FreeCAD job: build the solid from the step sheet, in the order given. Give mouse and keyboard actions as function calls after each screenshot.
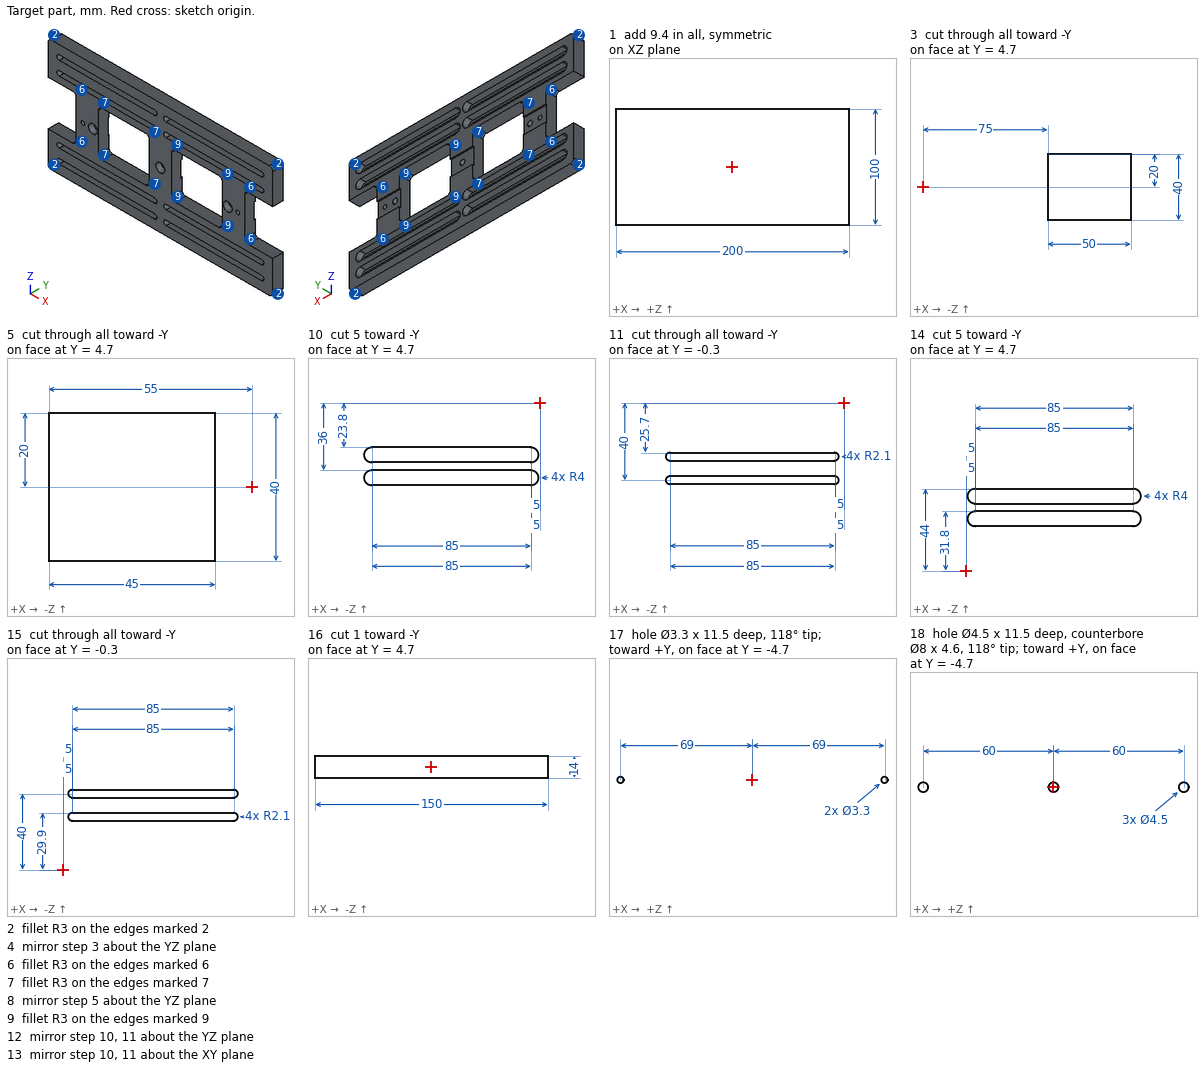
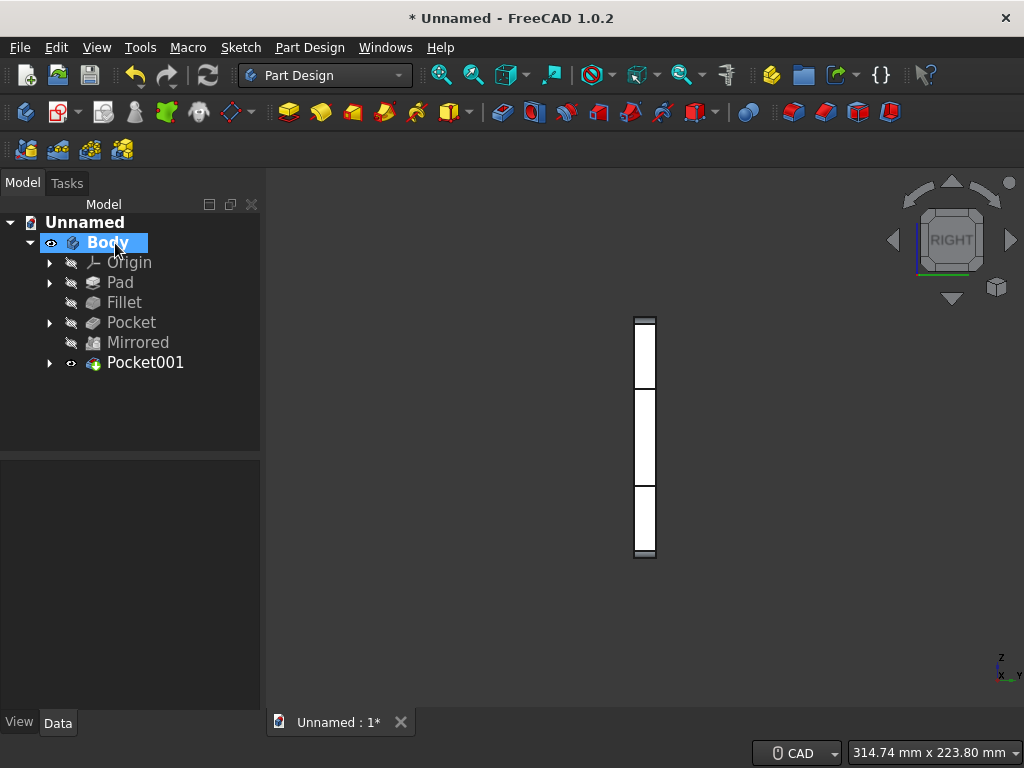
key(5)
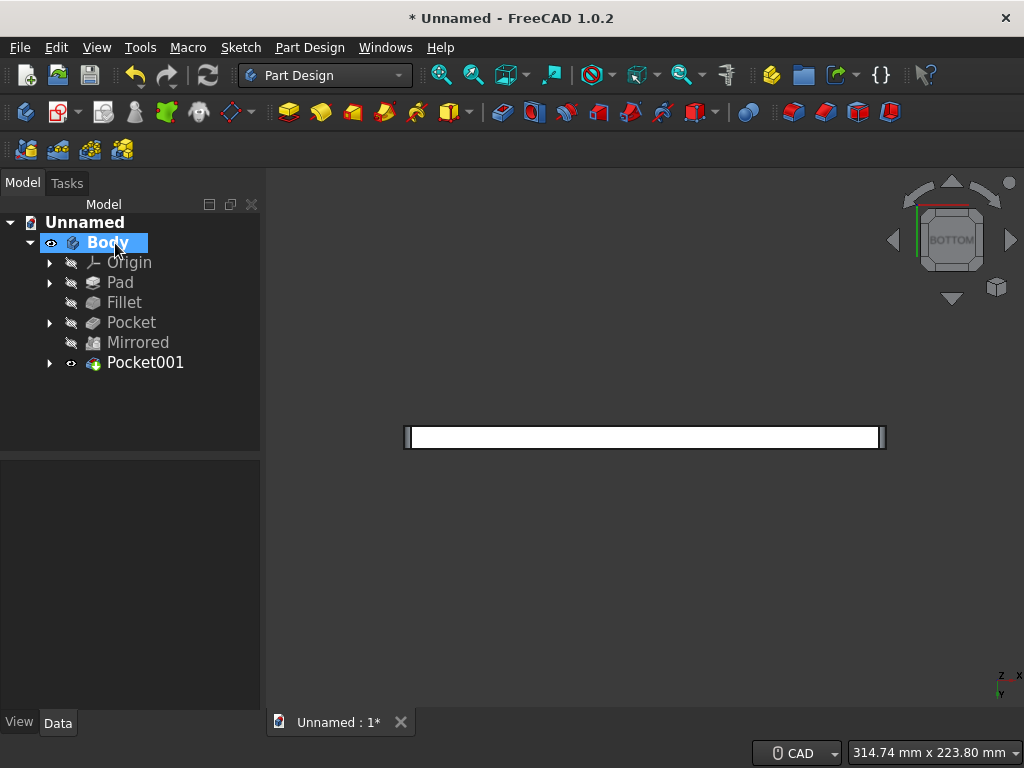
key(4)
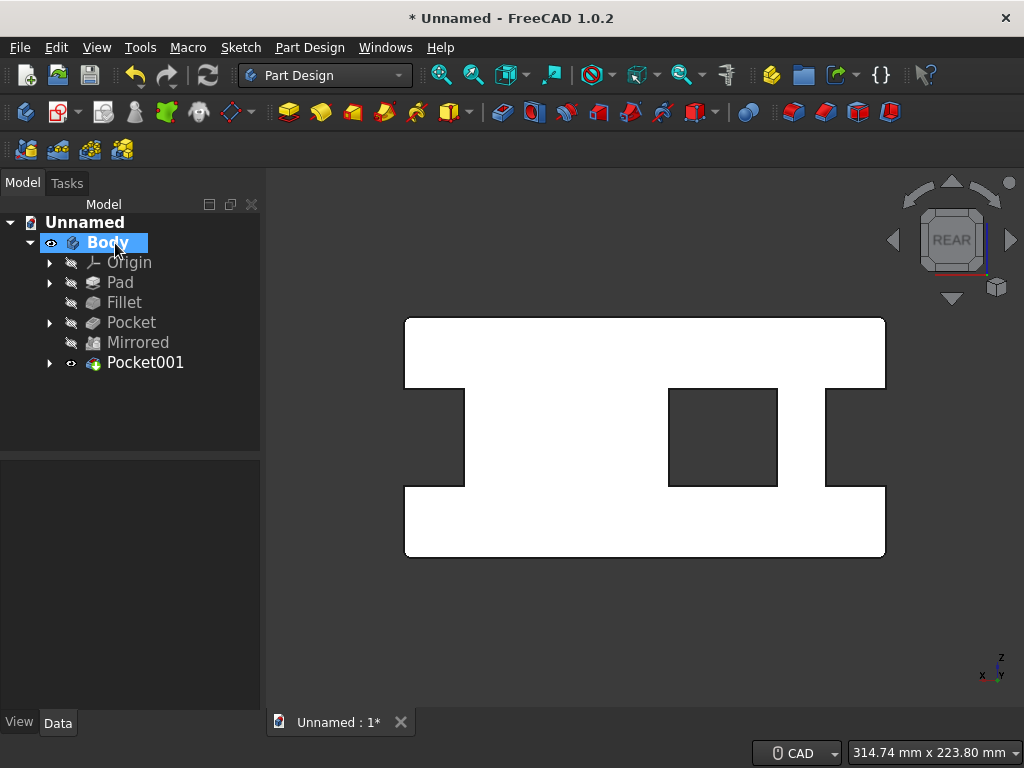
key(6)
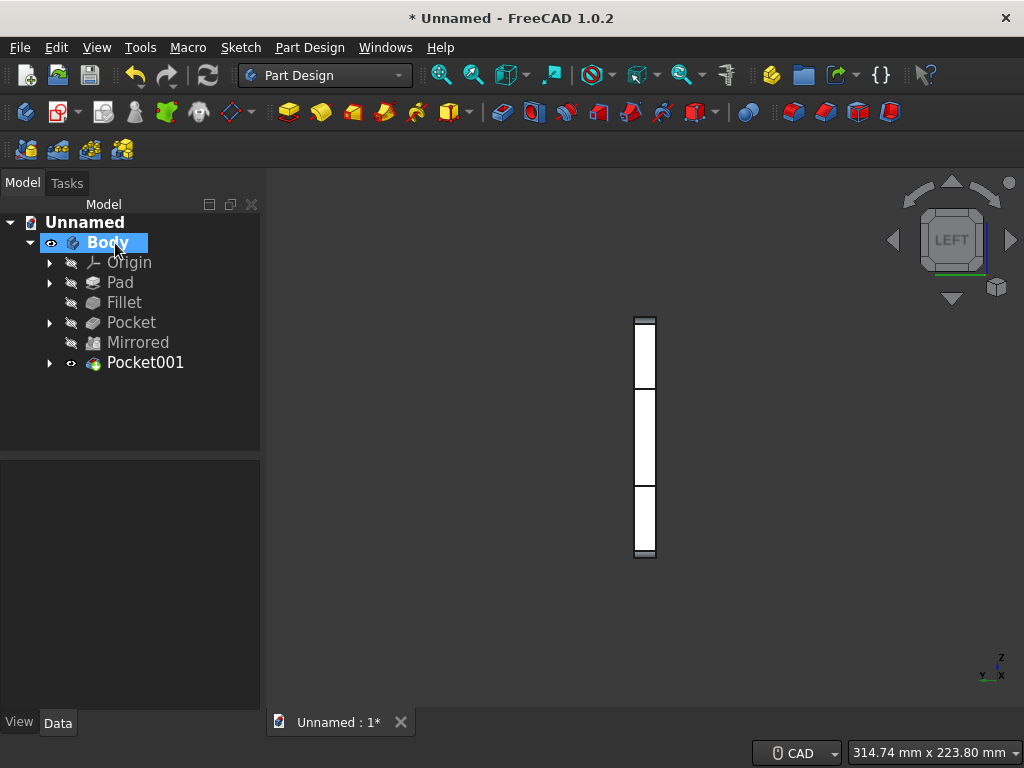
click(442, 76)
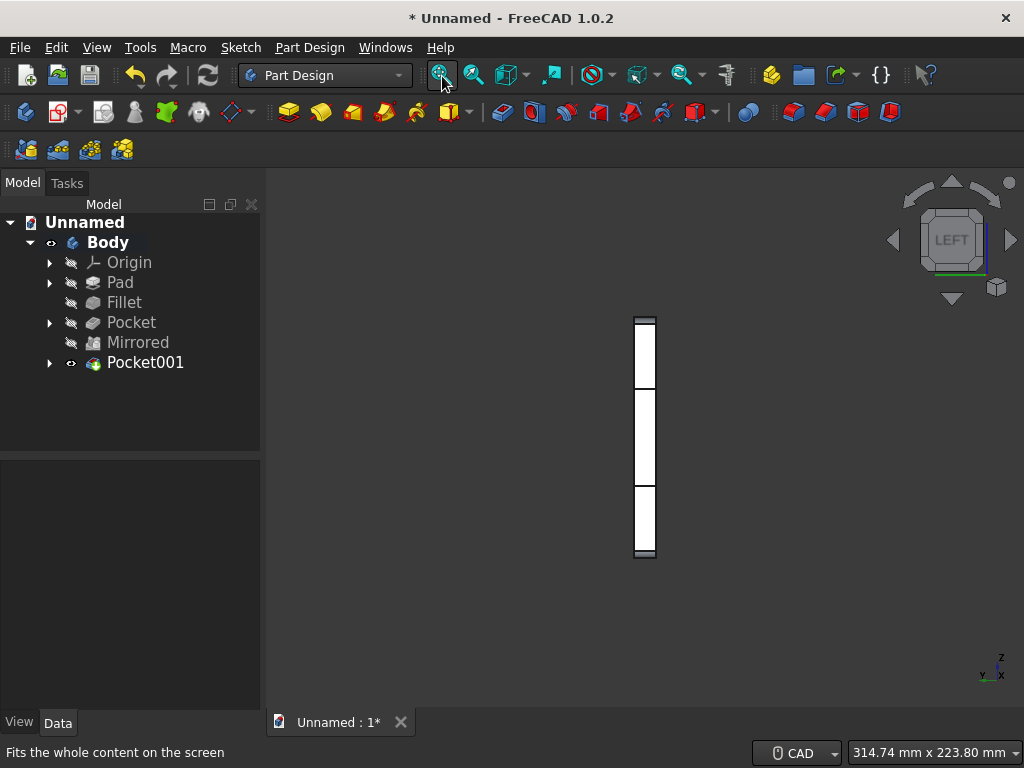
key(v)
key(3)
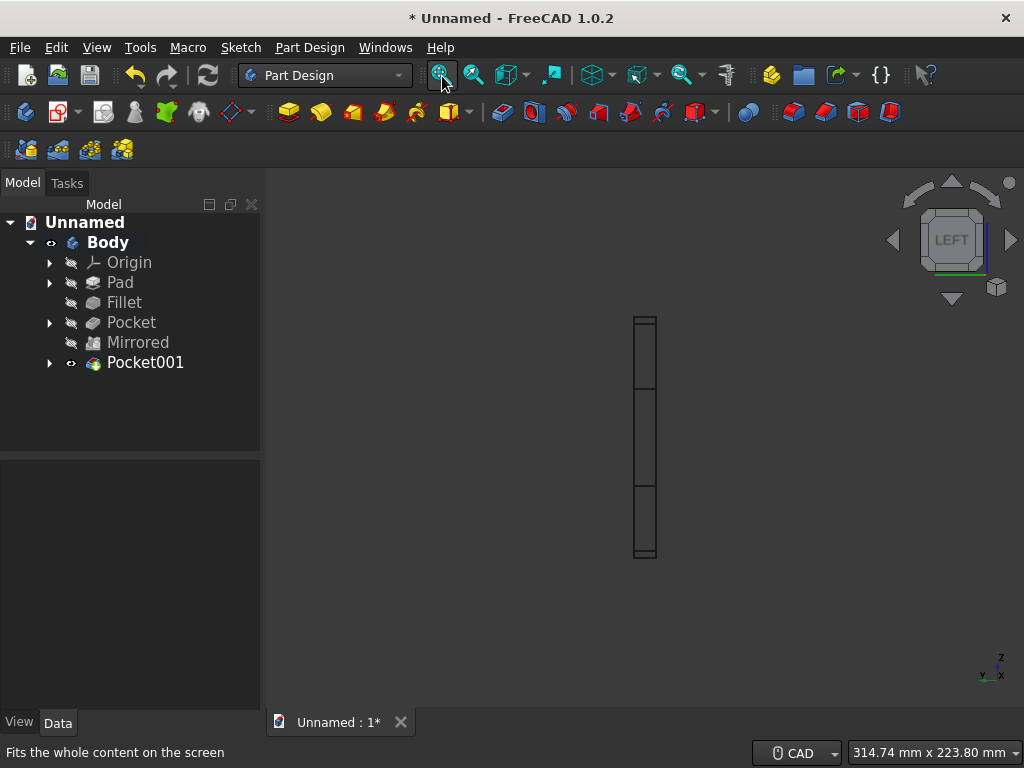
key(0)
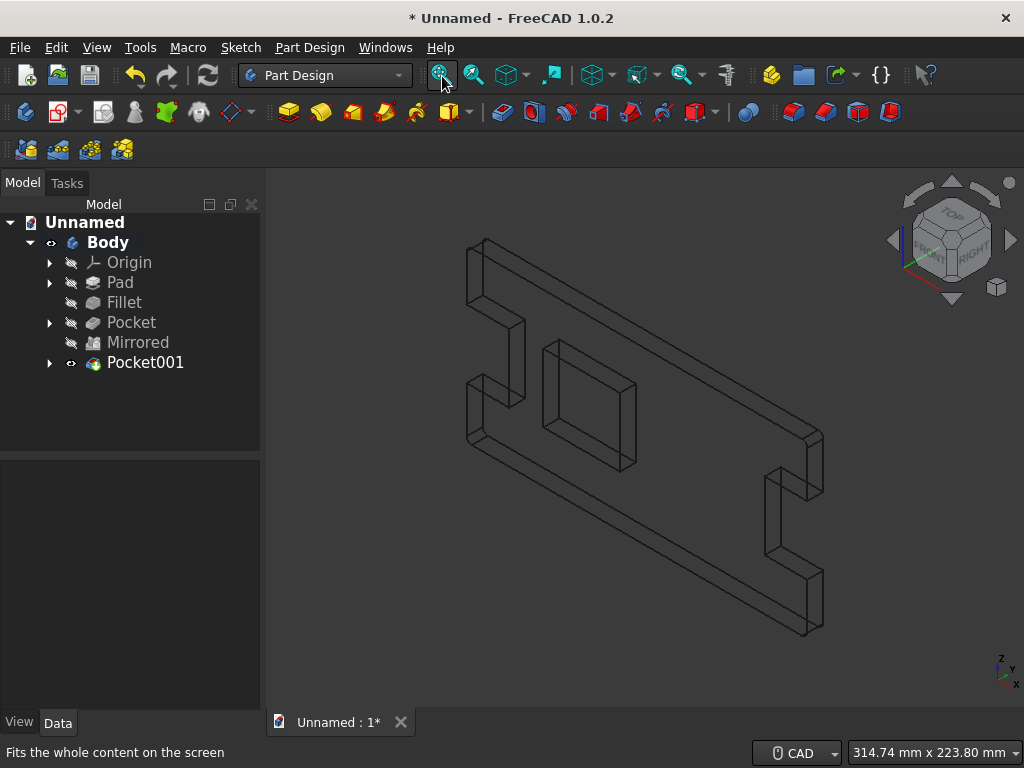
click(773, 550)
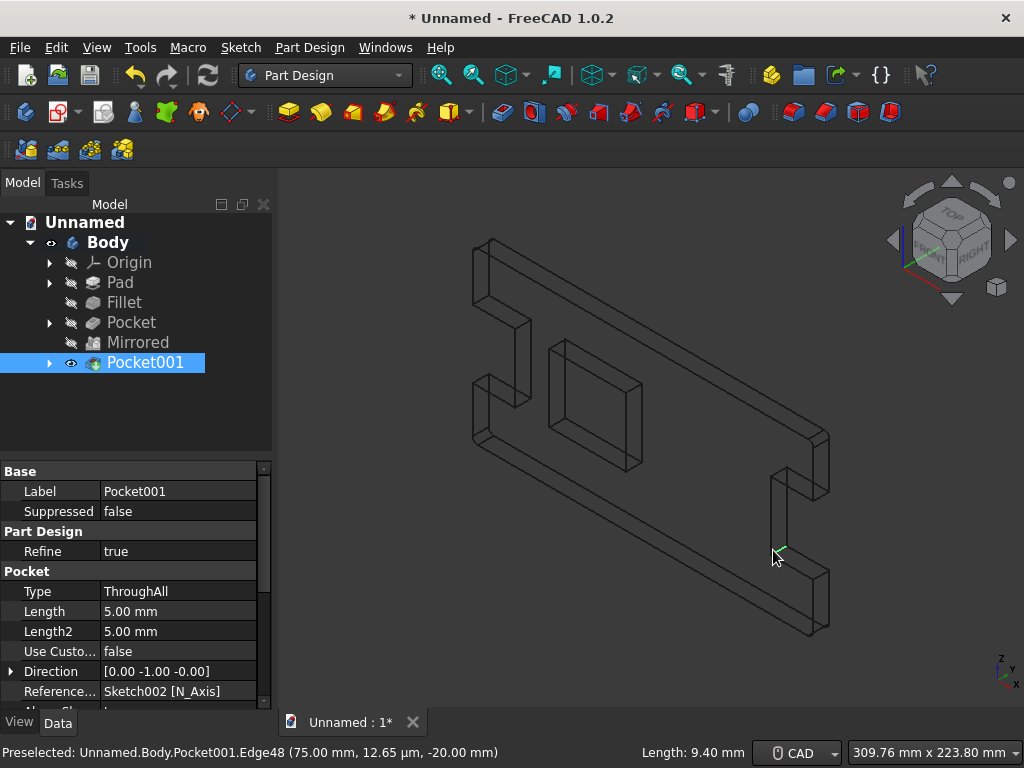
click(779, 471, ctrl)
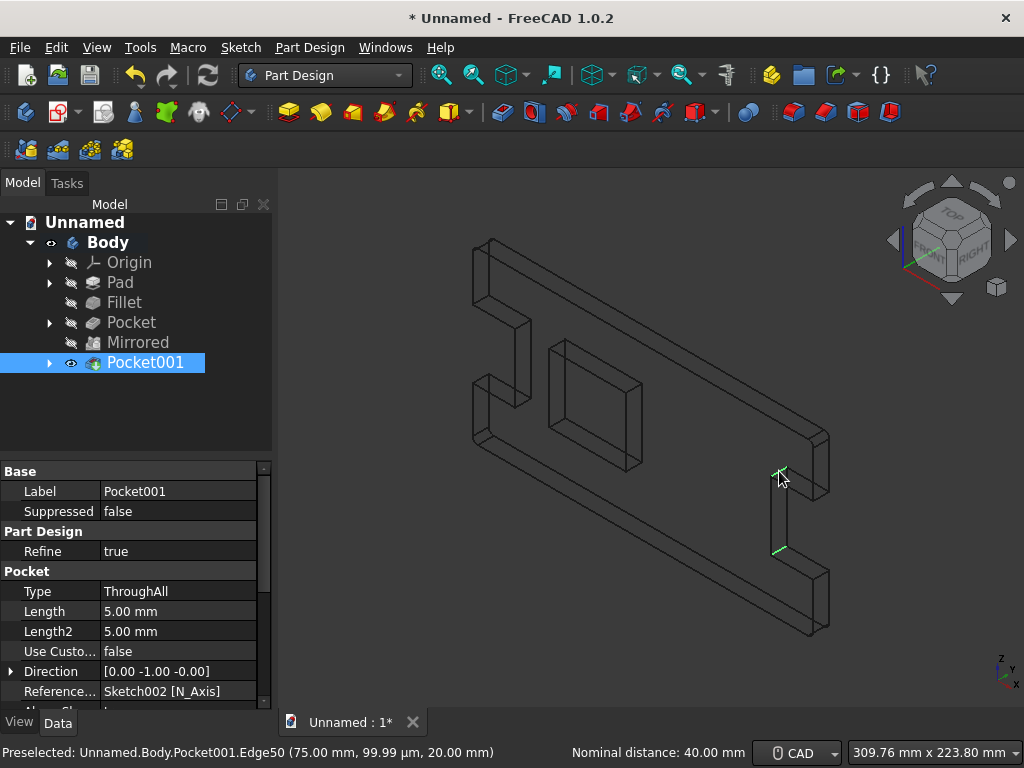
click(523, 323, ctrl)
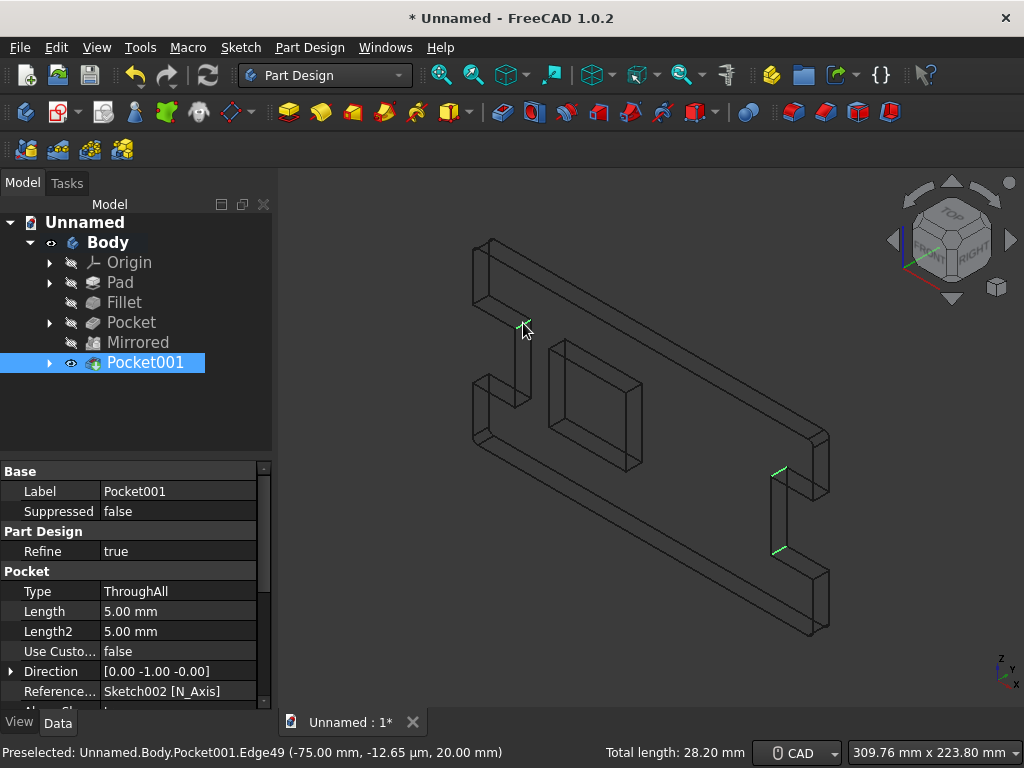
click(523, 402, ctrl)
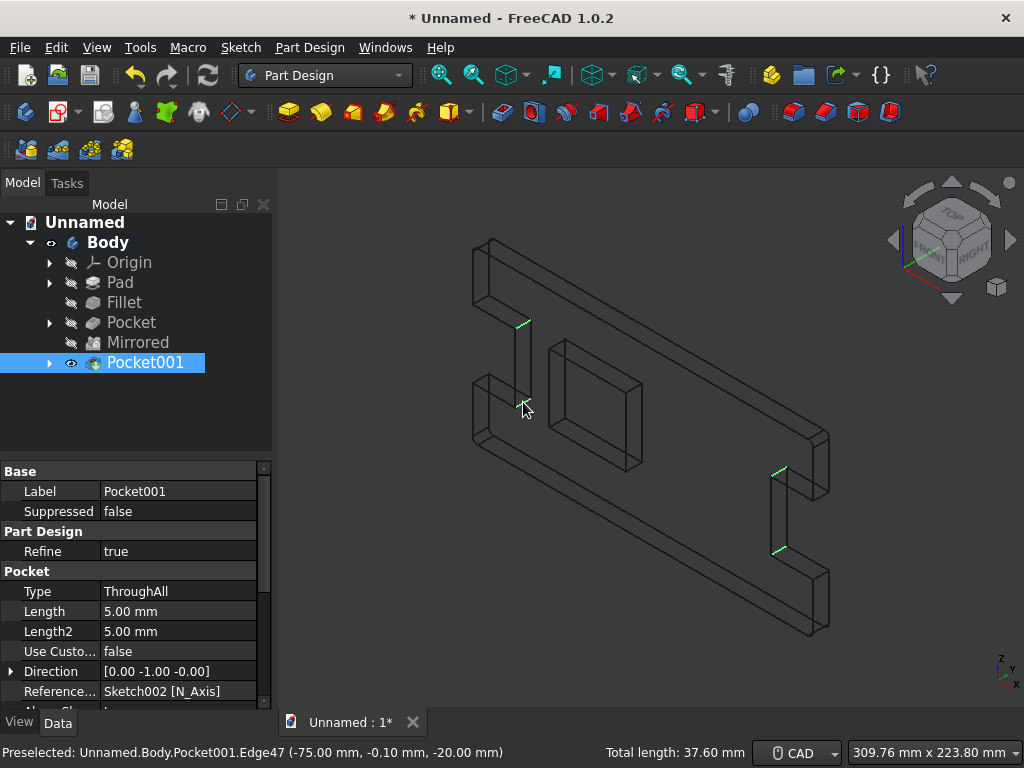
key(v)
key(1)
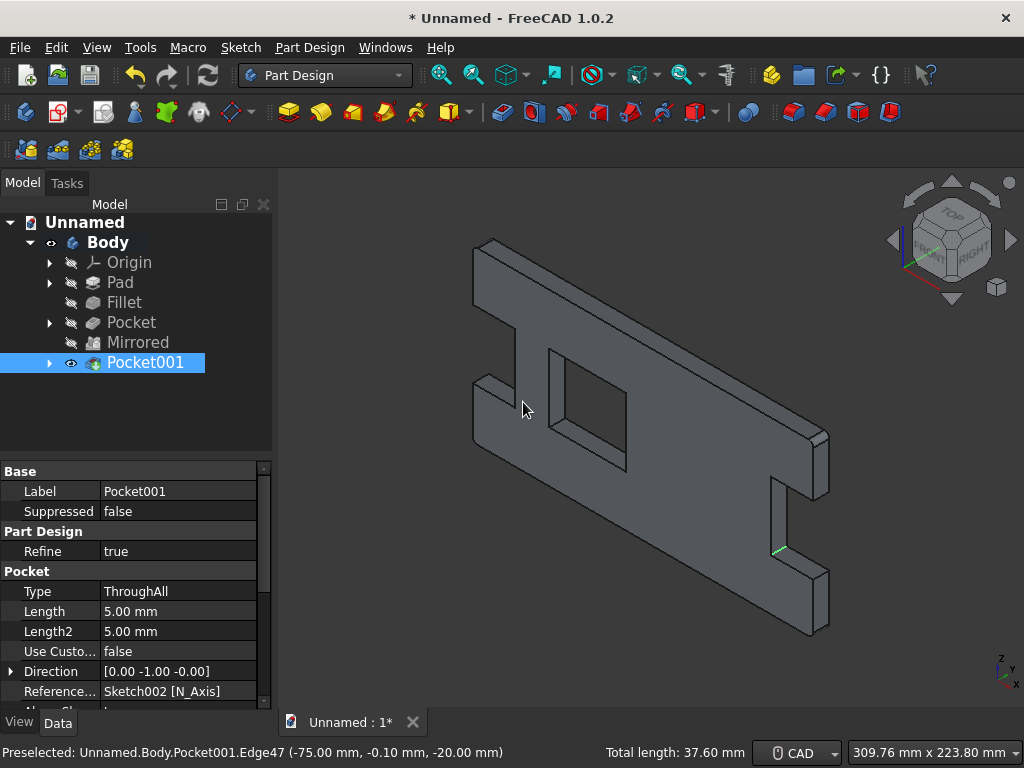
click(794, 112)